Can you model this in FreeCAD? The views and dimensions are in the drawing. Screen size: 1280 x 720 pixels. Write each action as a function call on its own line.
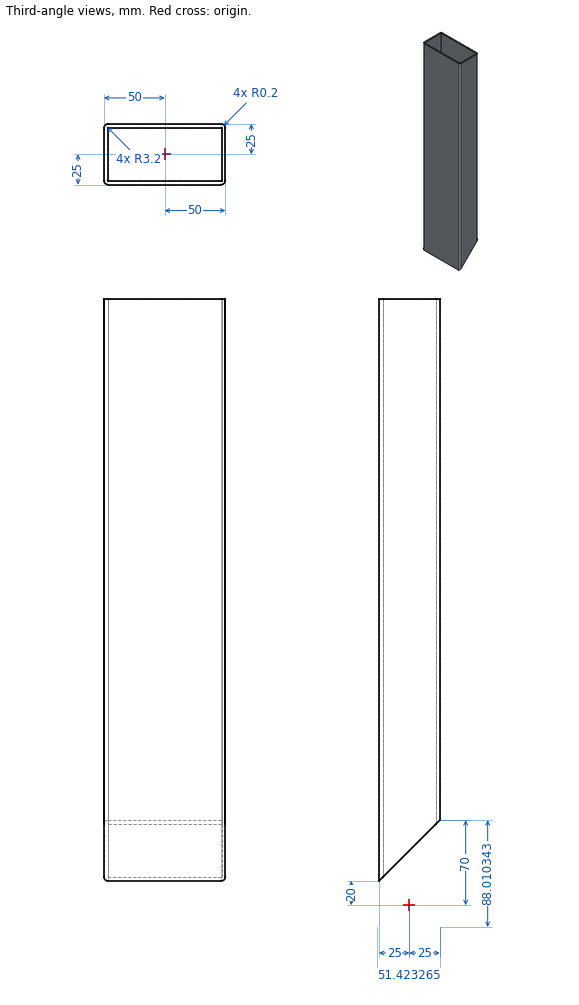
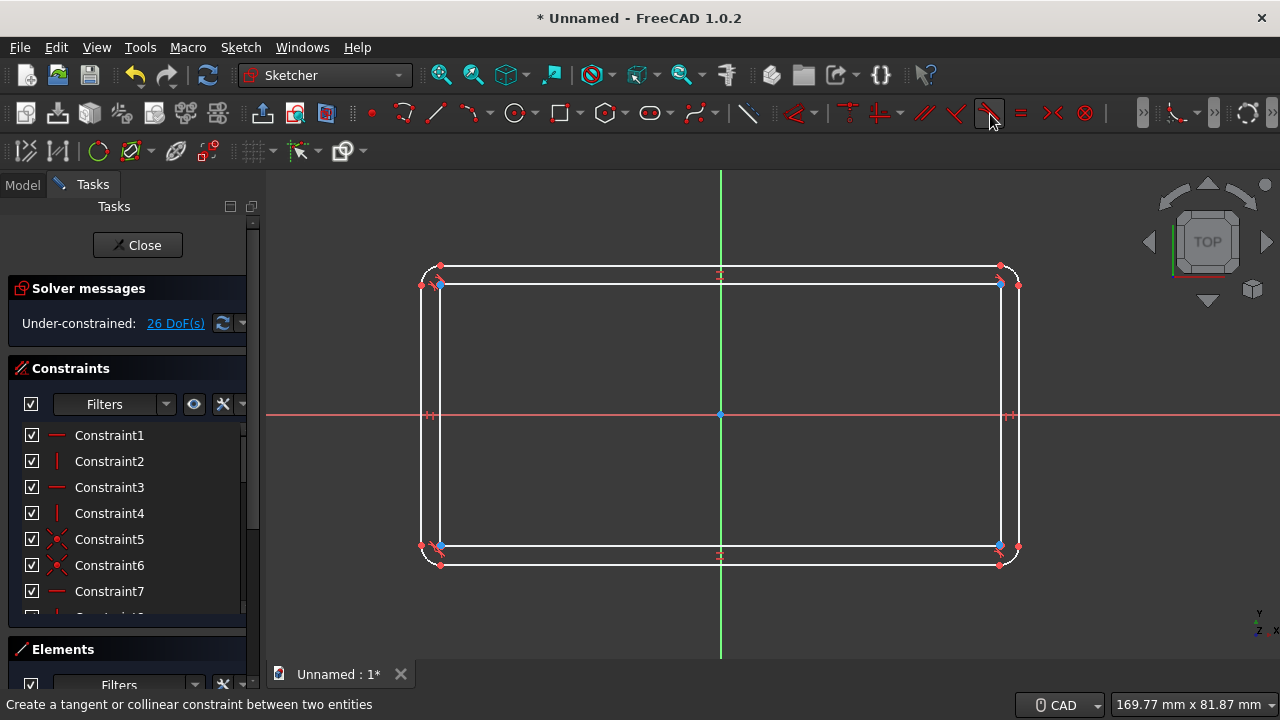
click(1019, 468)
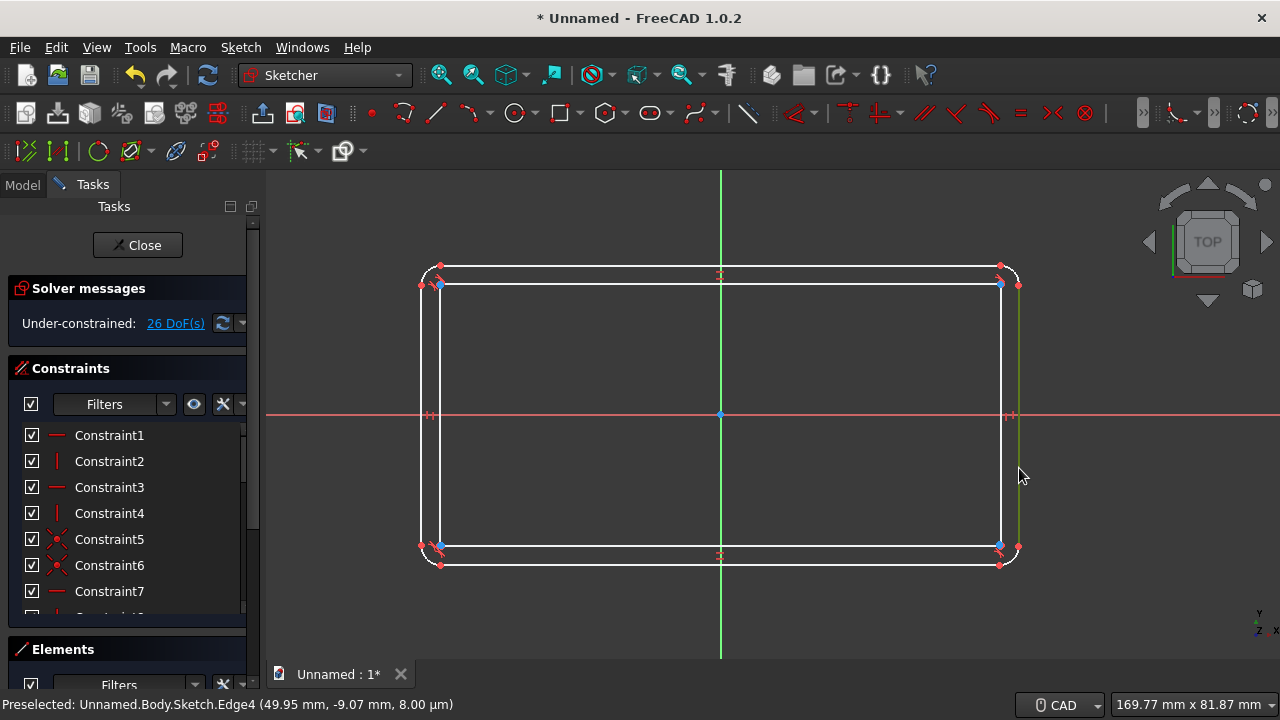
click(1013, 560)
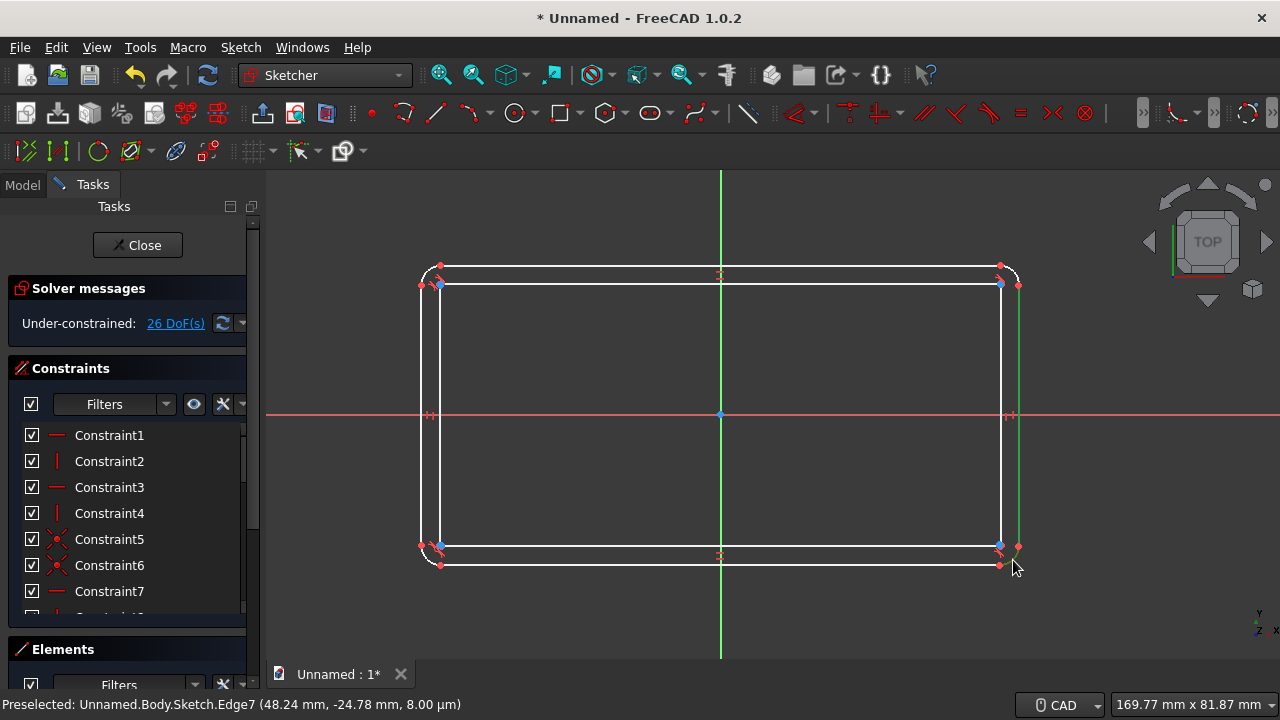
click(990, 114)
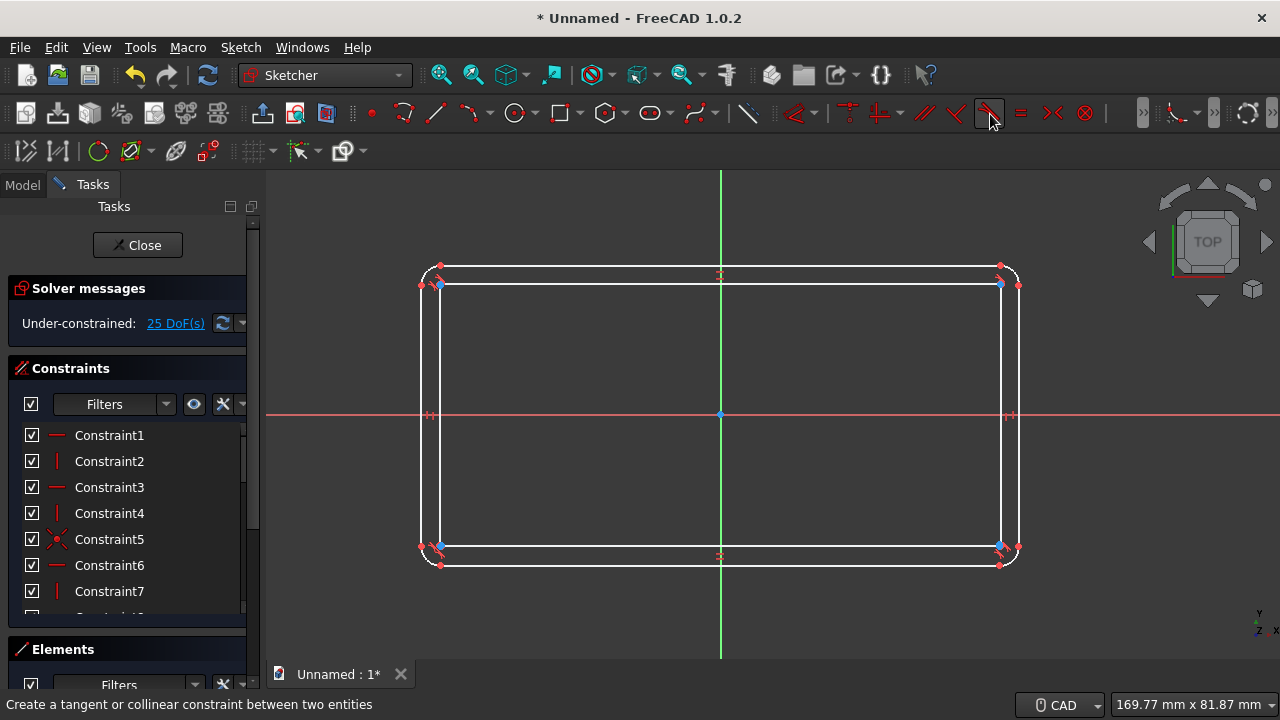
click(1019, 468)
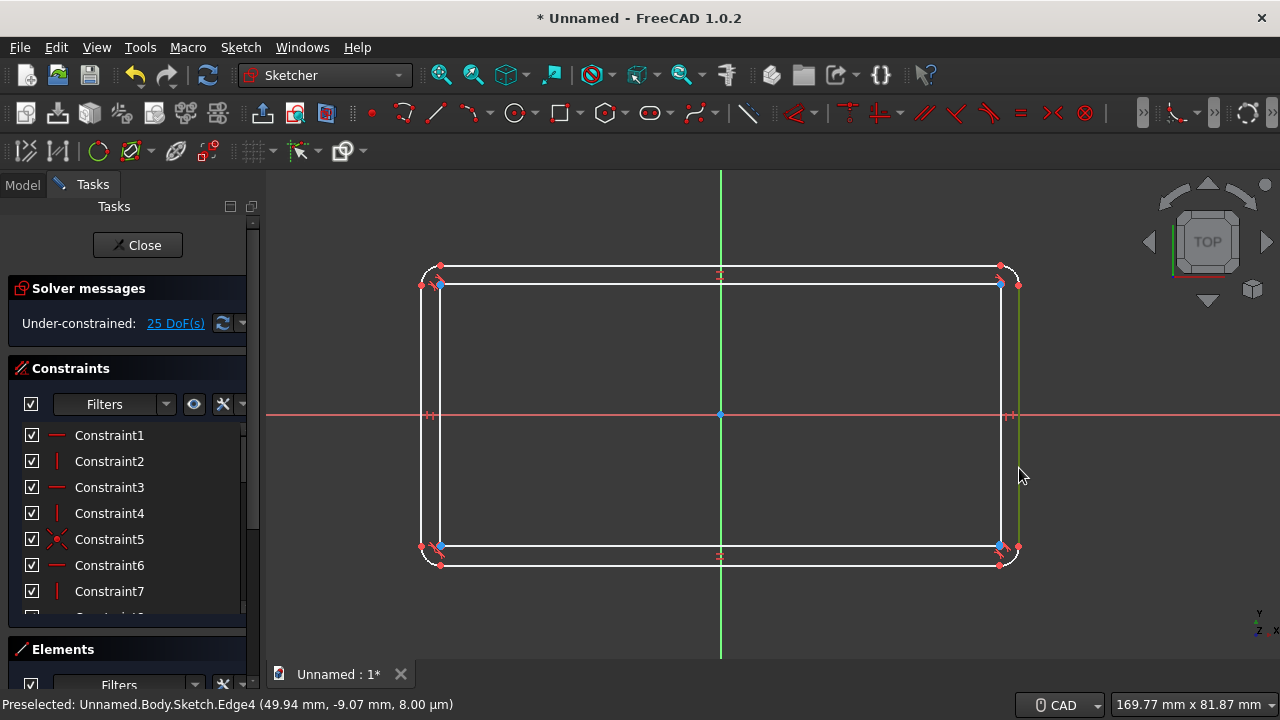
click(1014, 272)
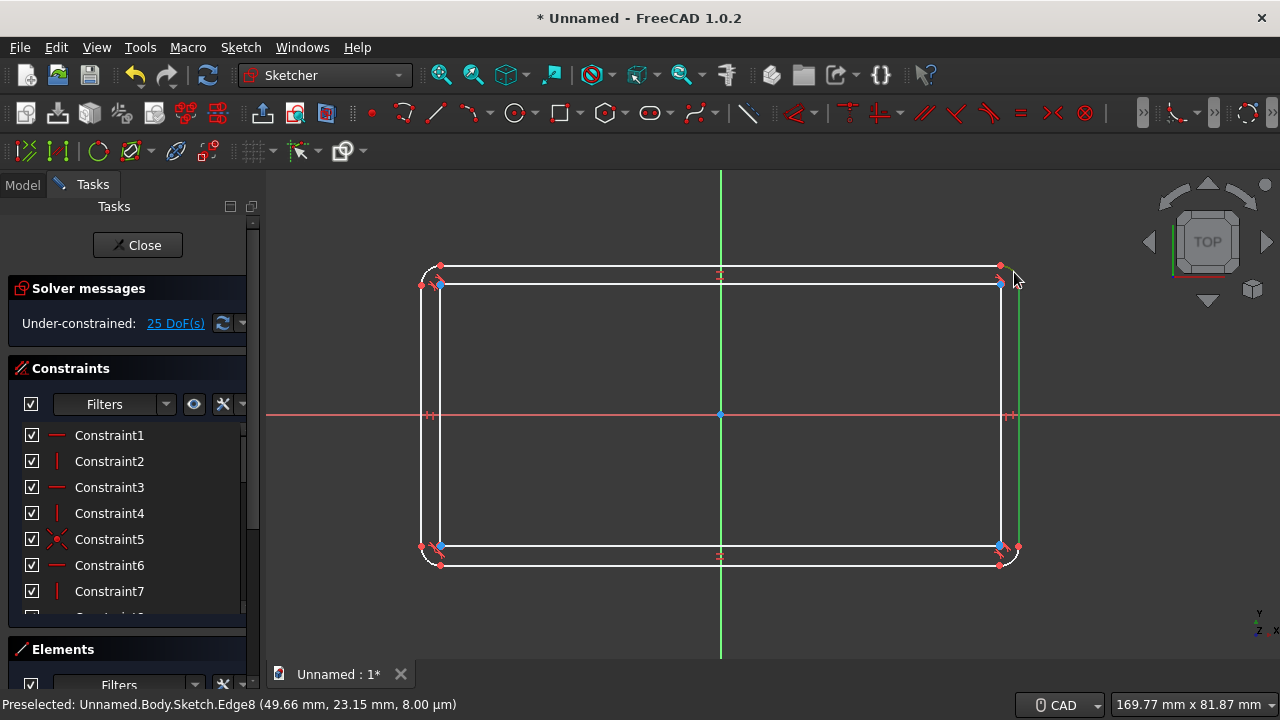
click(990, 114)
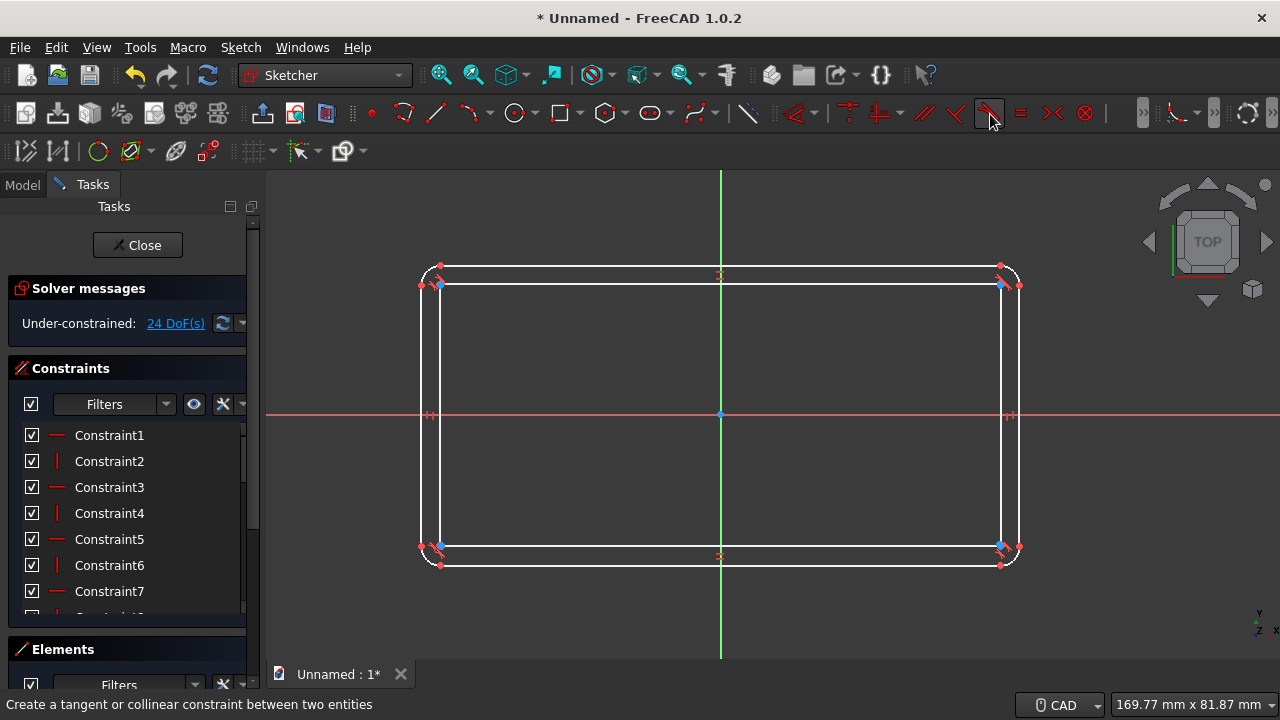
click(609, 284)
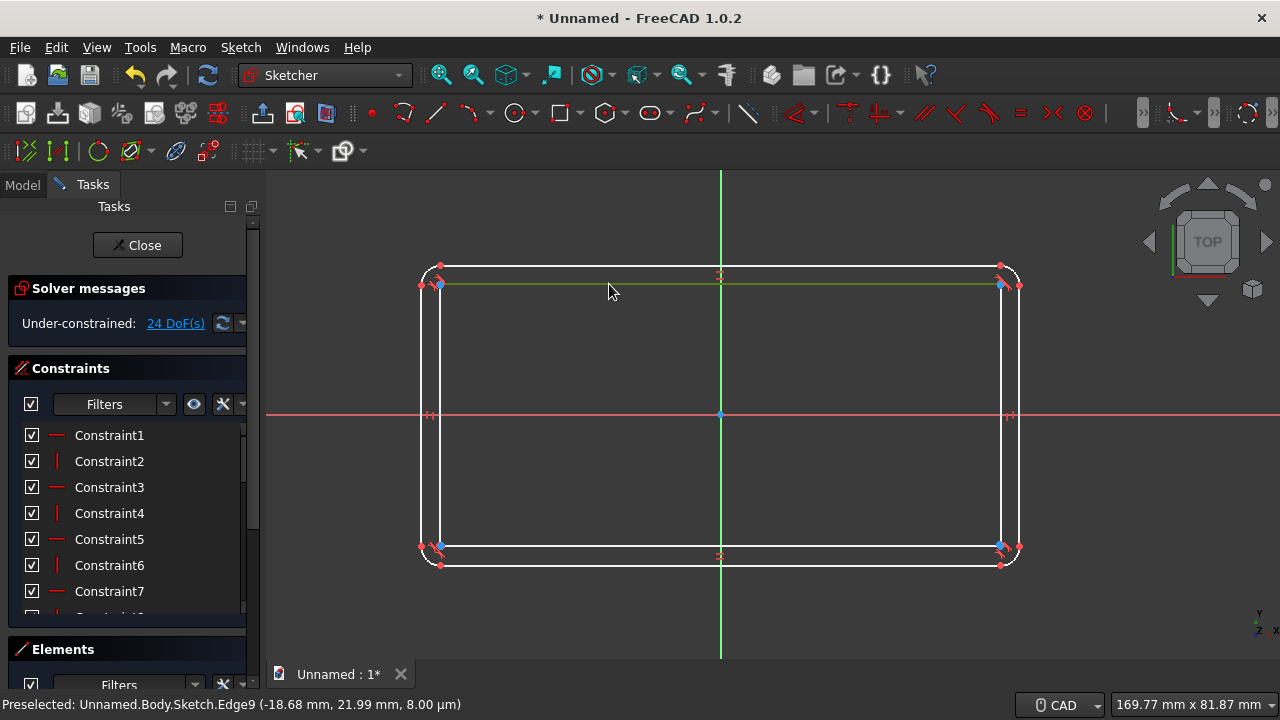
scroll(1001, 284, up, 13)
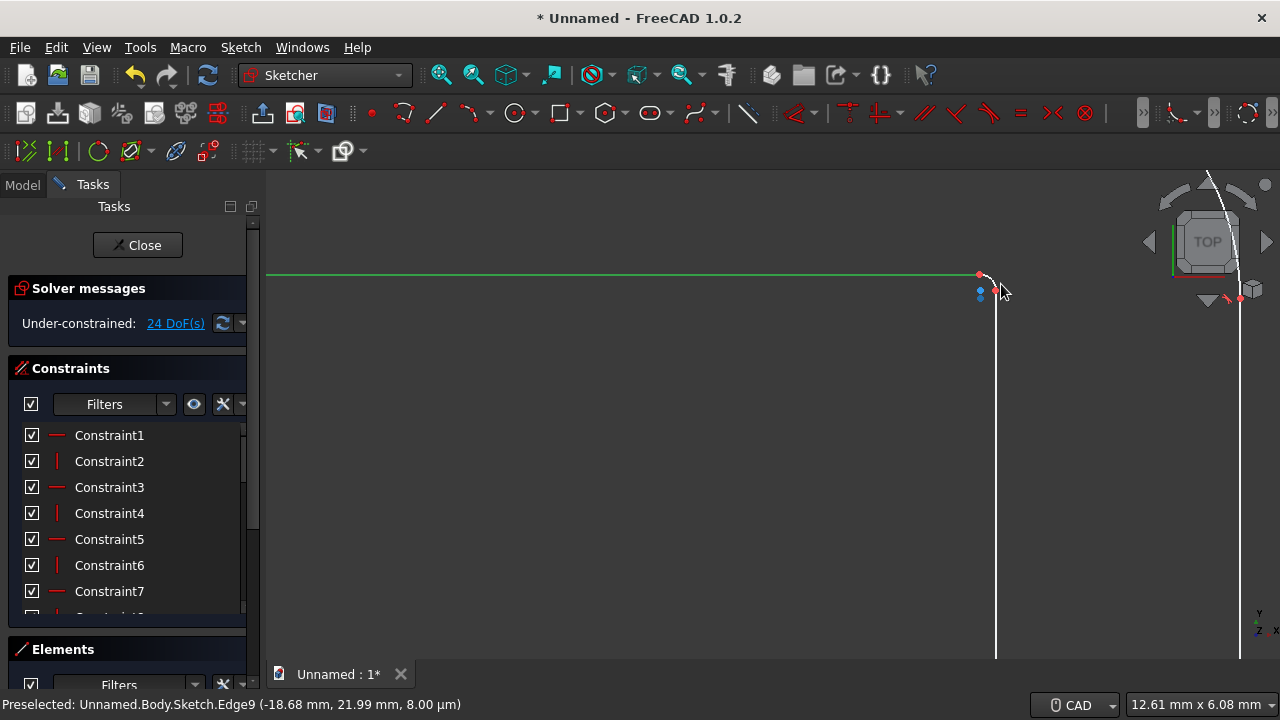
click(991, 279)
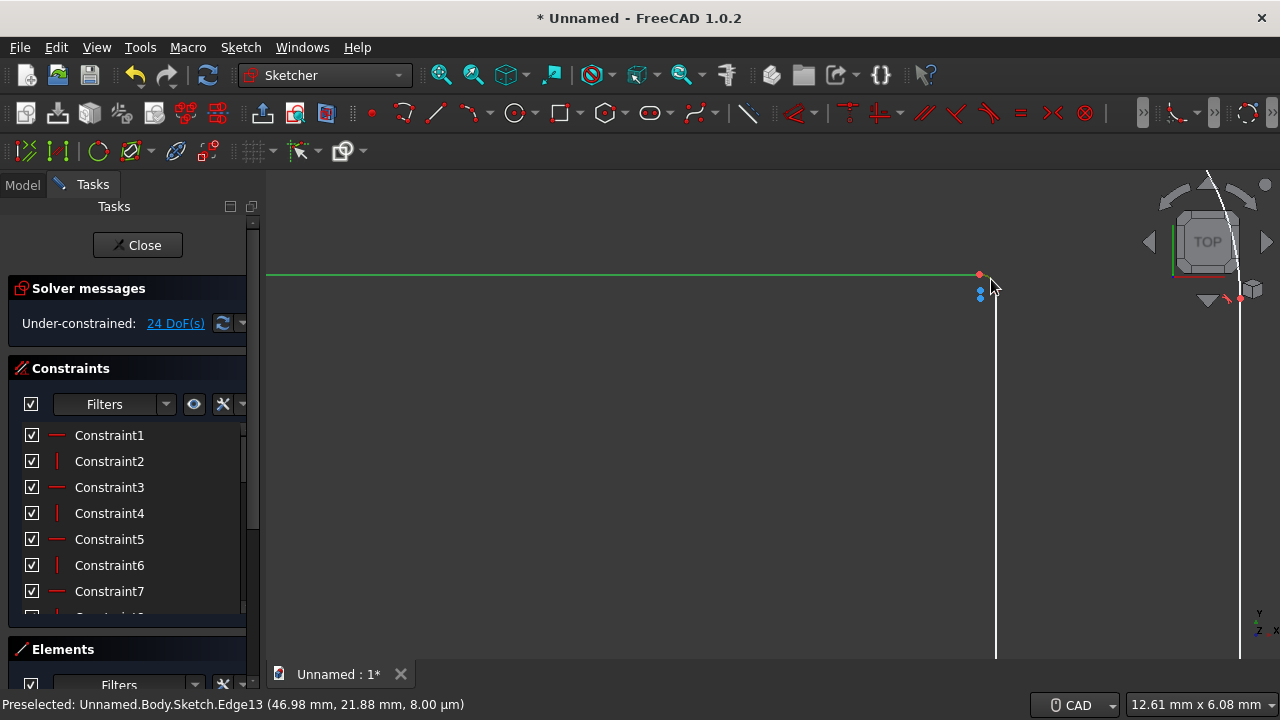
click(990, 114)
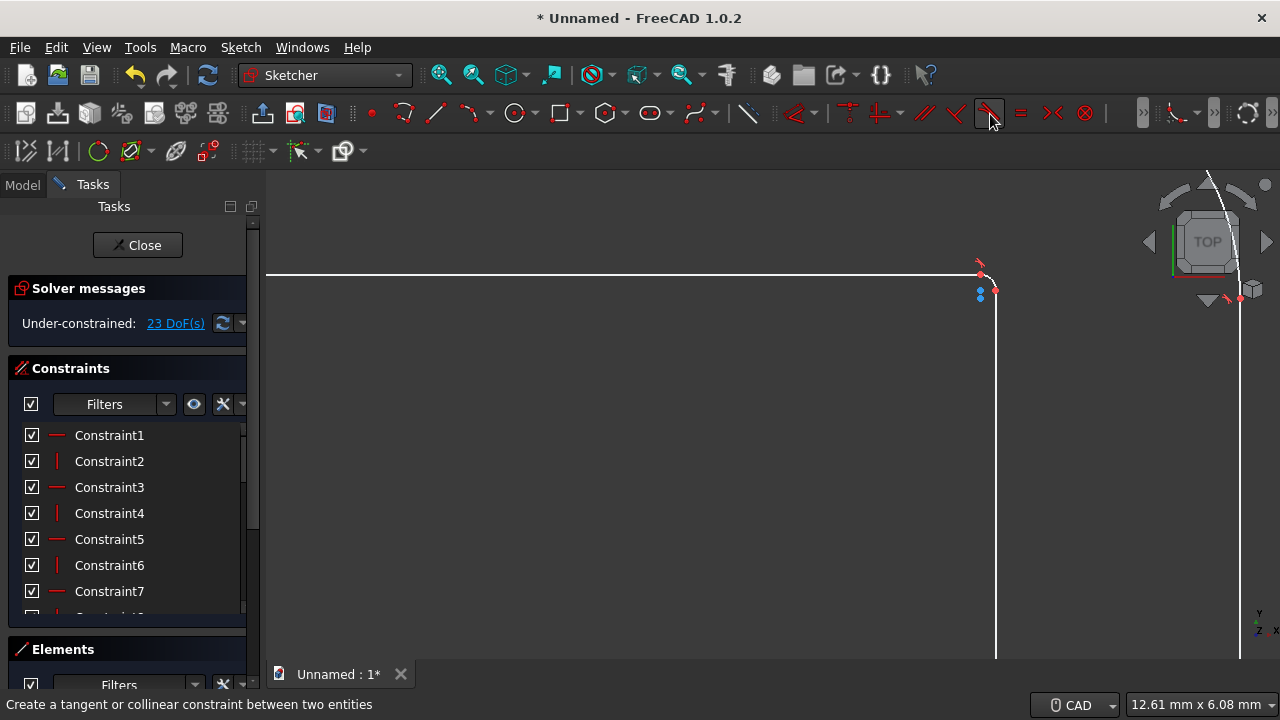
scroll(984, 284, down, 13)